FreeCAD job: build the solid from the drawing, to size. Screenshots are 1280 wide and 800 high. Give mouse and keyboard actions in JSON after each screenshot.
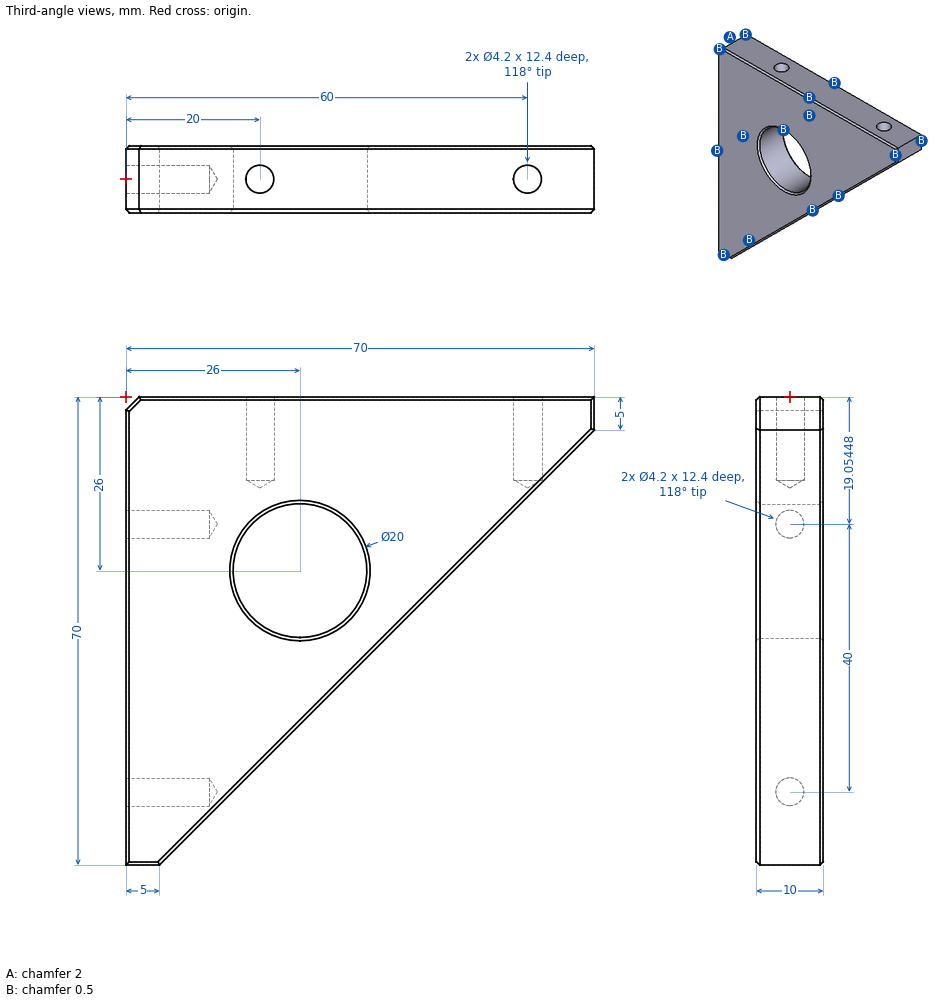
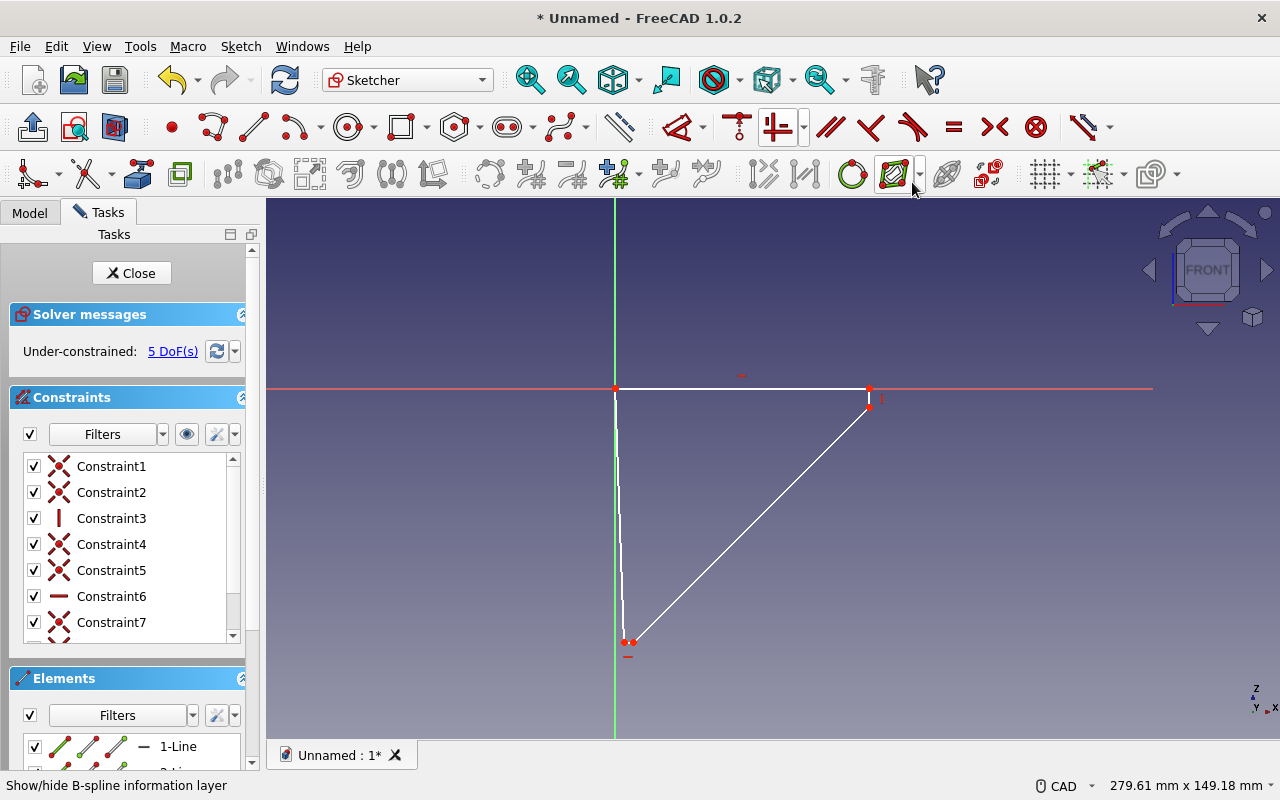
{"action": "left_click", "coordinate": [618, 465]}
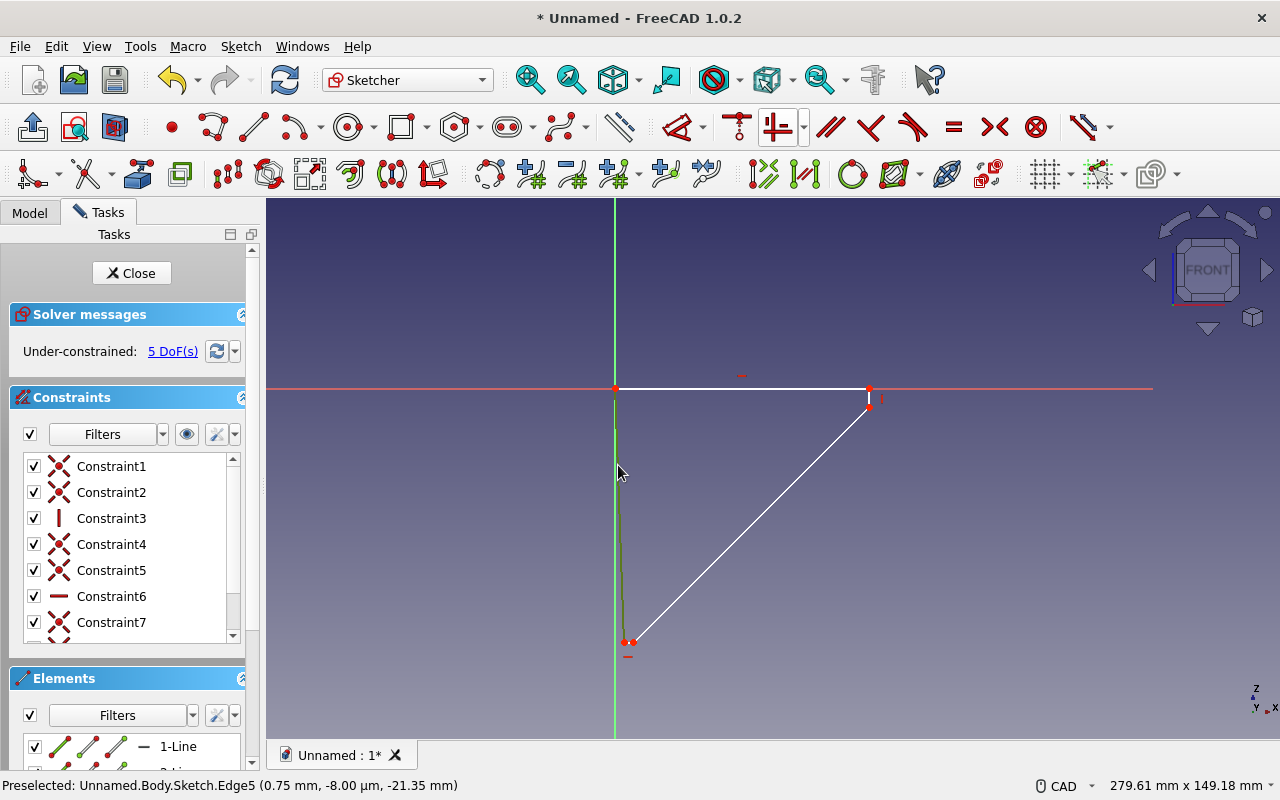
{"action": "left_click", "coordinate": [804, 128]}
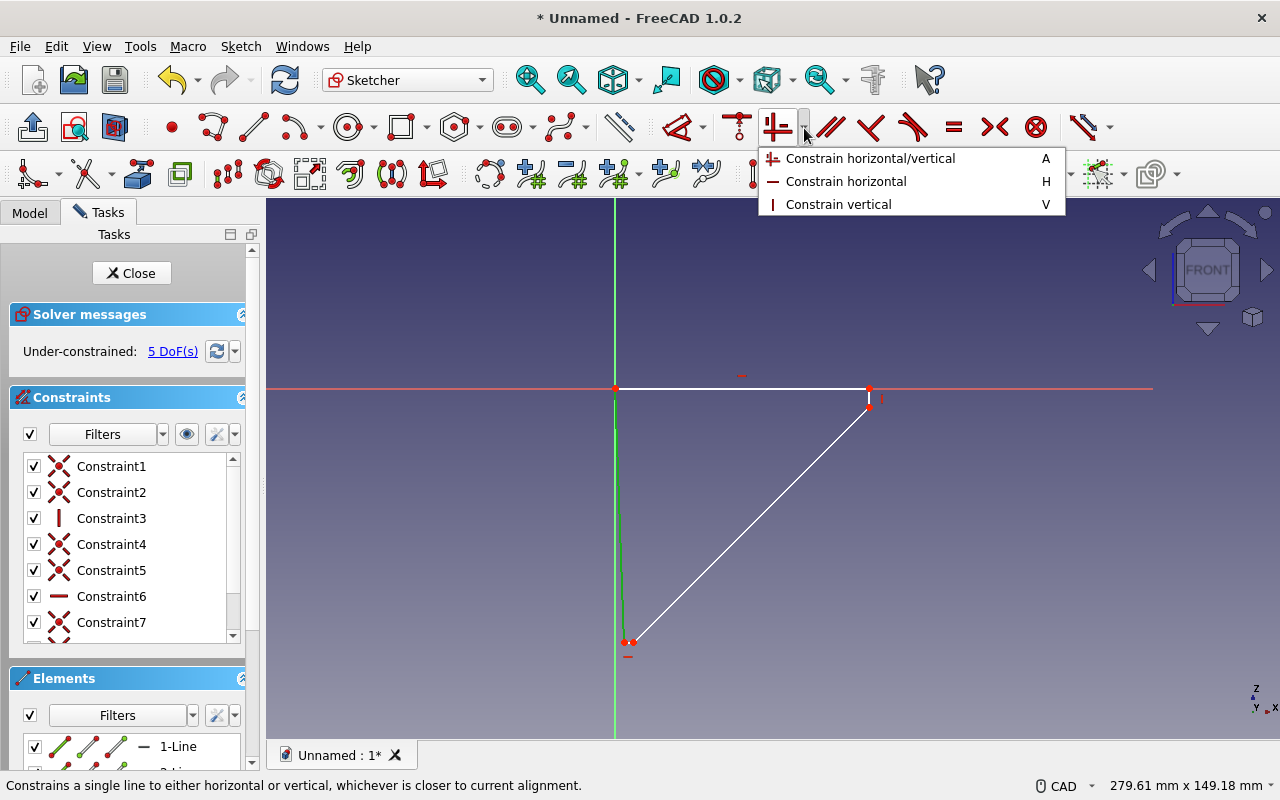
{"action": "left_click", "coordinate": [912, 204]}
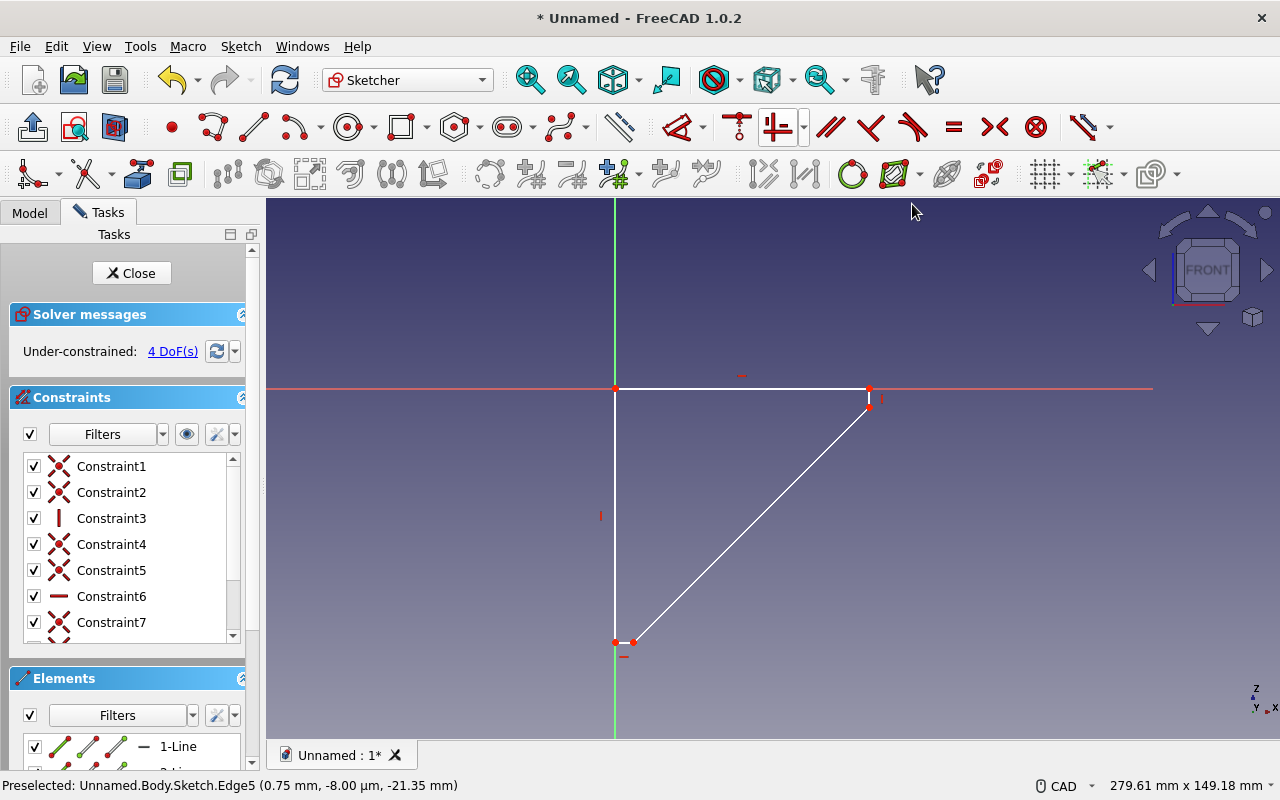
{"action": "scroll", "coordinate": [869, 398], "scroll_direction": "up", "scroll_amount": 4}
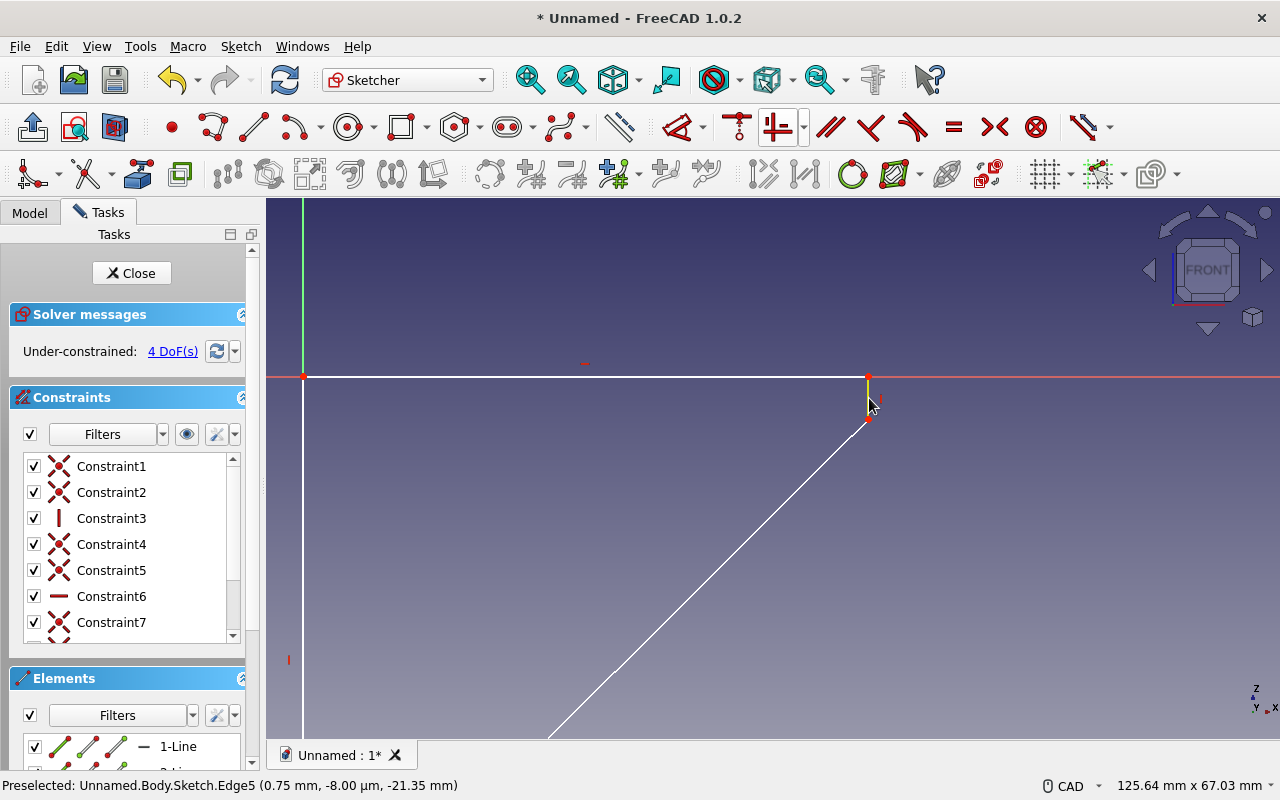
{"action": "left_click", "coordinate": [868, 398]}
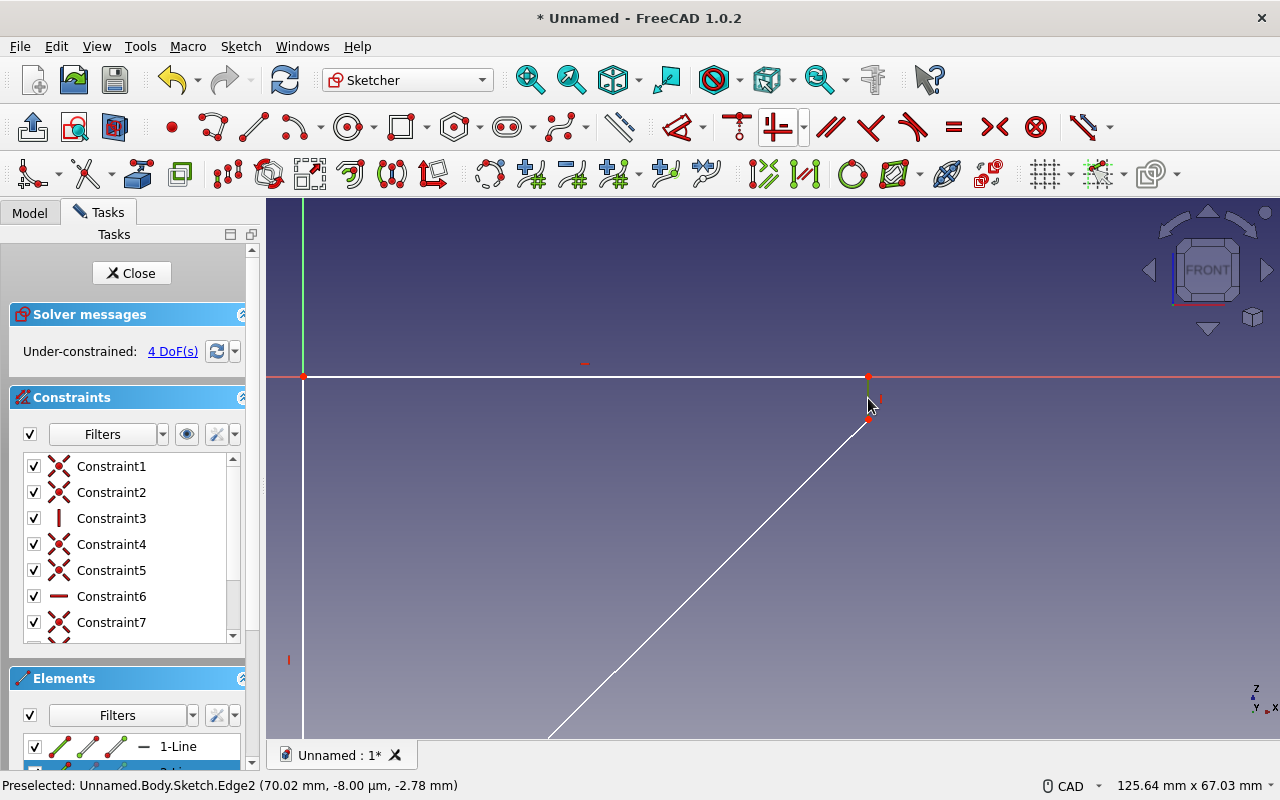
{"action": "left_click", "coordinate": [702, 128]}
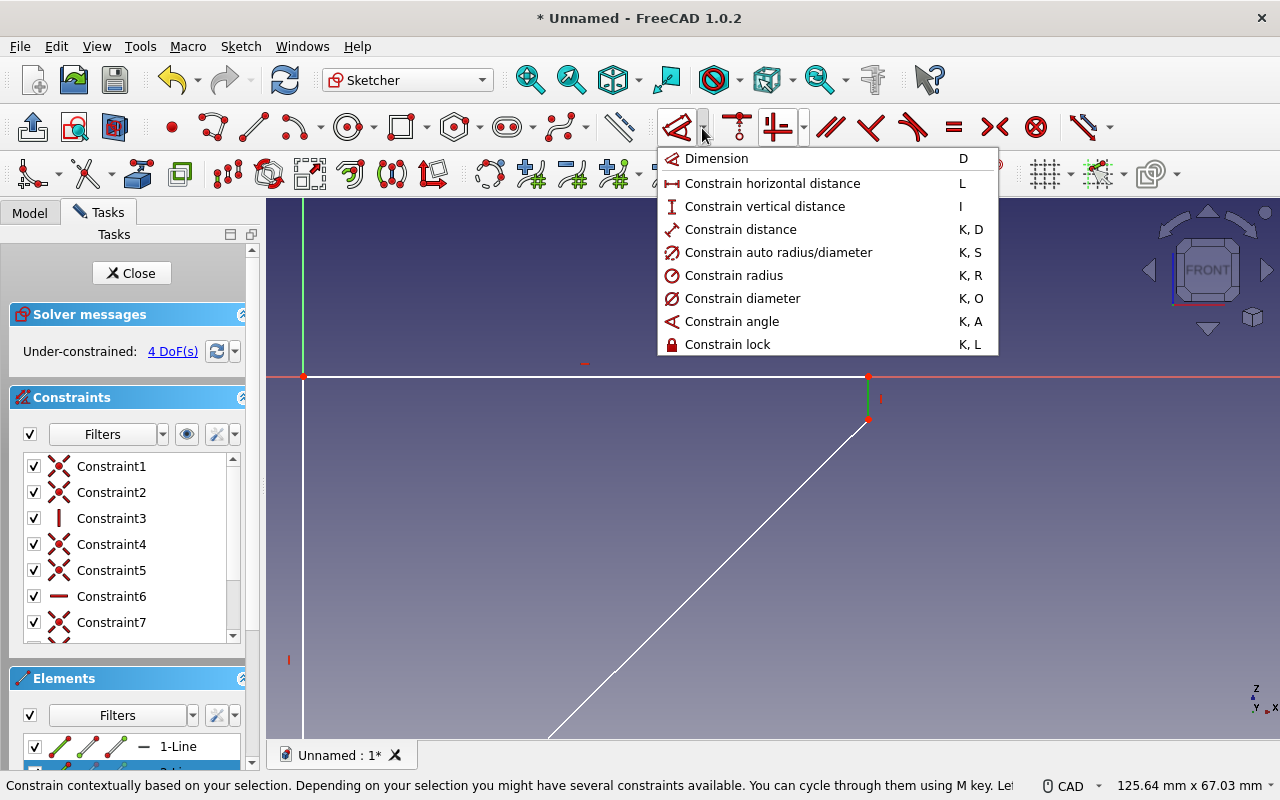
{"action": "left_click", "coordinate": [828, 206]}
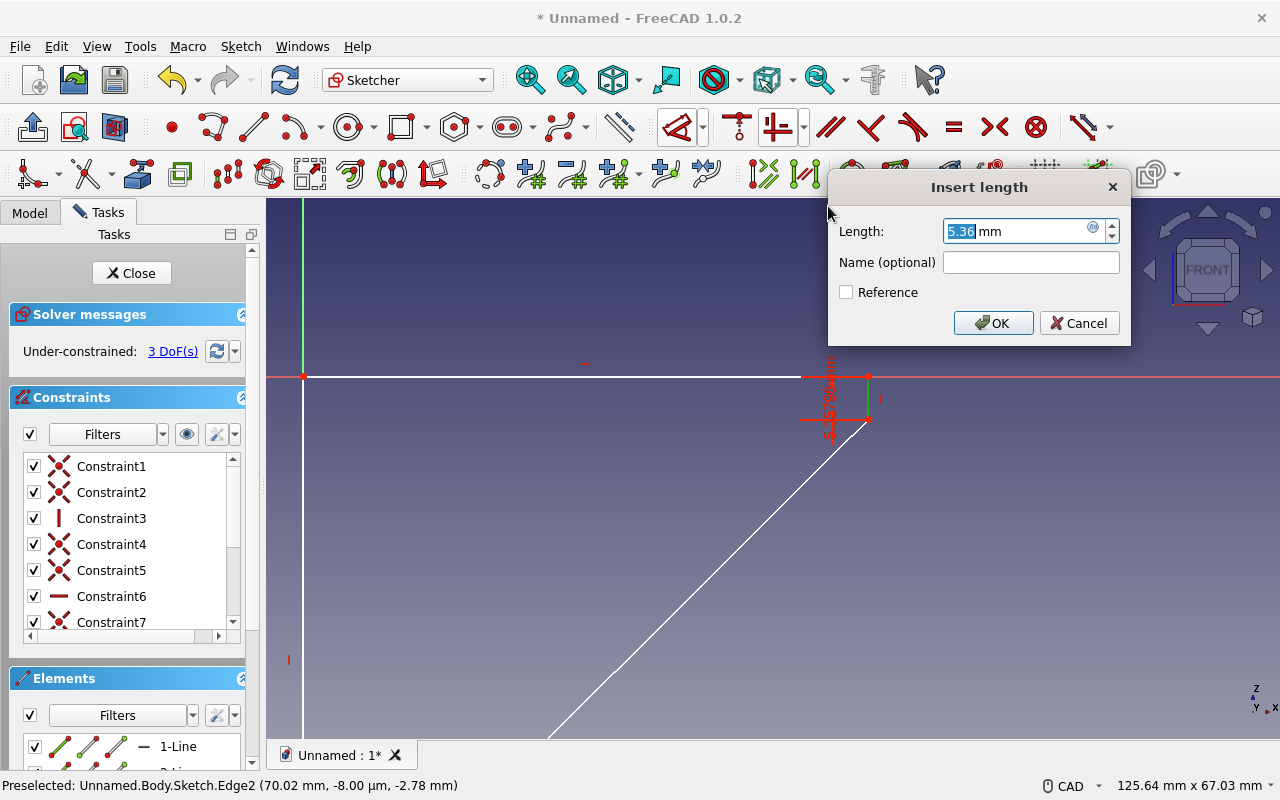
{"action": "type", "text": "5"}
{"action": "key", "text": "Return"}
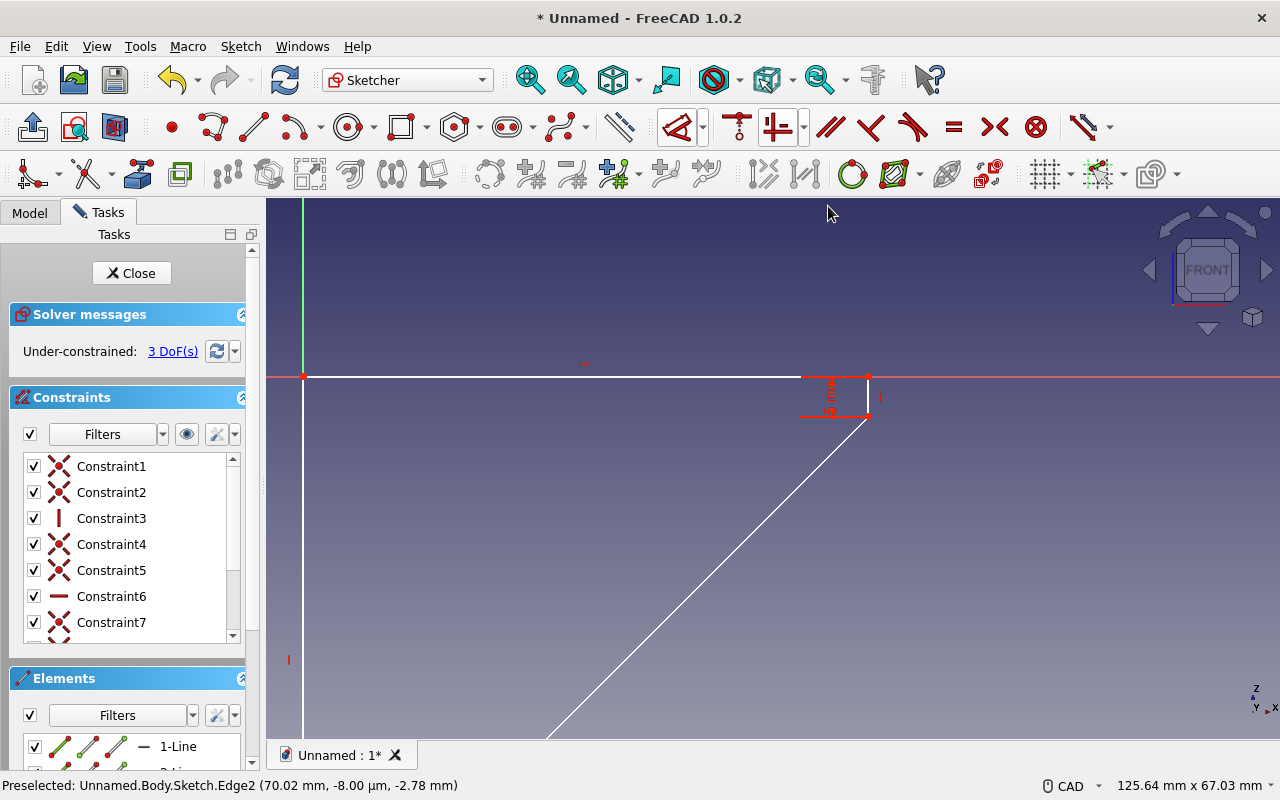
{"action": "scroll", "coordinate": [849, 237], "scroll_direction": "down", "scroll_amount": 3}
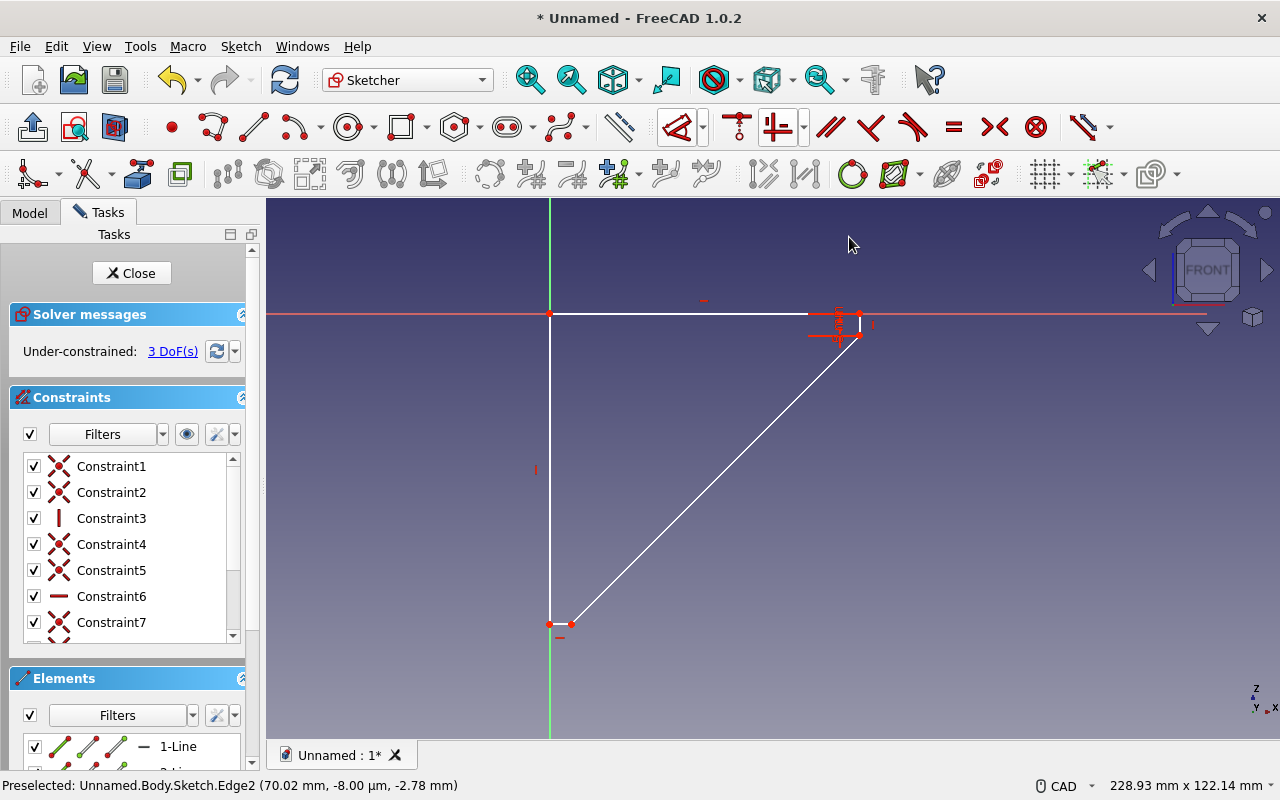
{"action": "scroll", "coordinate": [565, 624], "scroll_direction": "up", "scroll_amount": 4}